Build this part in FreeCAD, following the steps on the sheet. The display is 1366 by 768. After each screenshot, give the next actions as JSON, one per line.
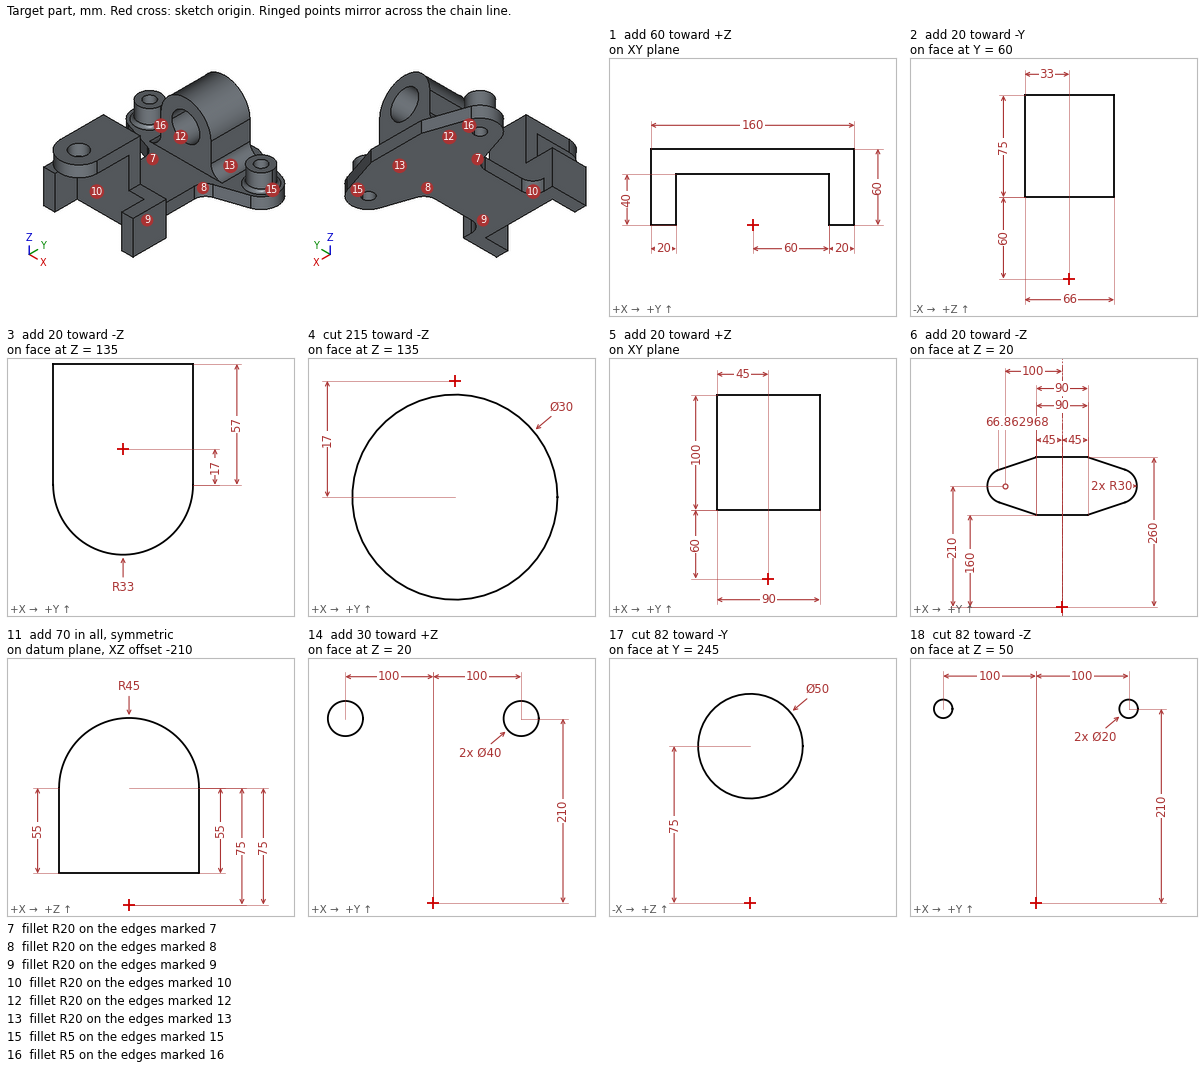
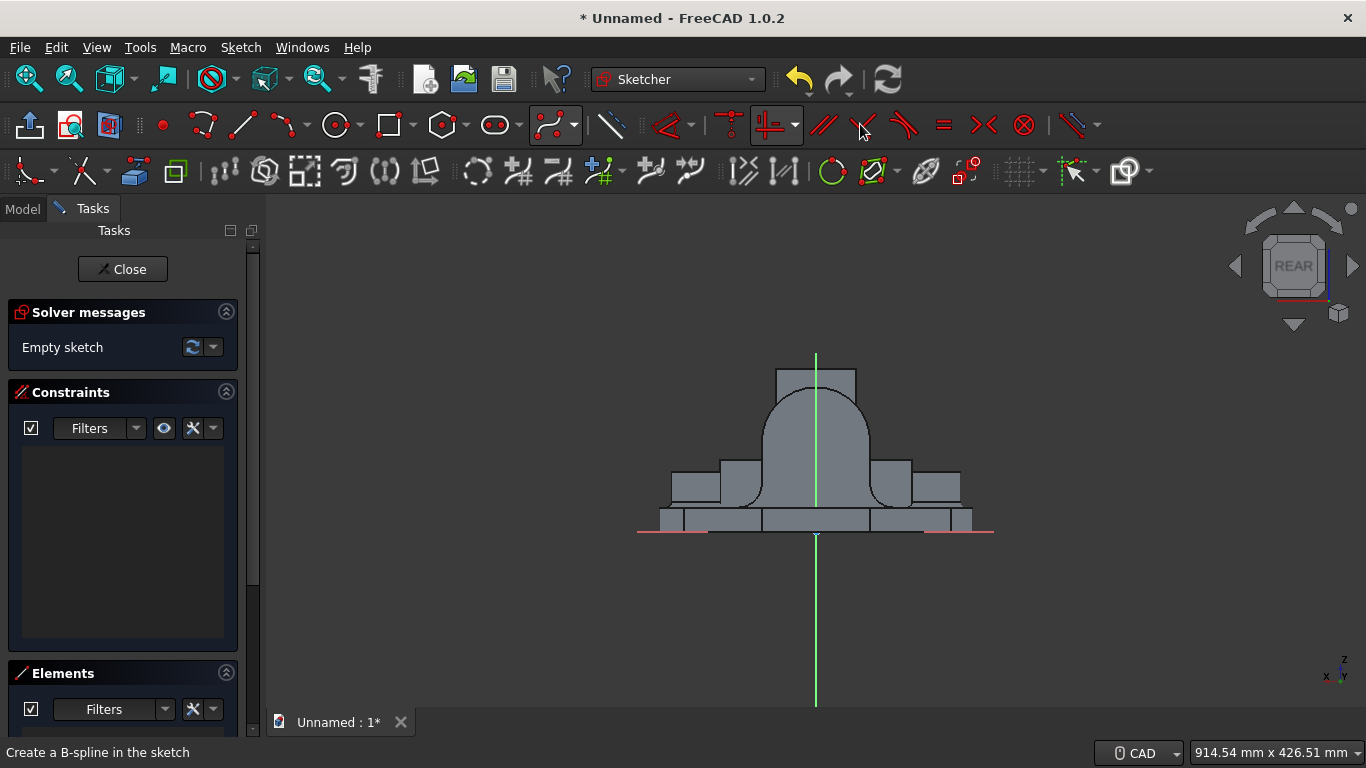
{"action": "left_click", "coordinate": [110, 126]}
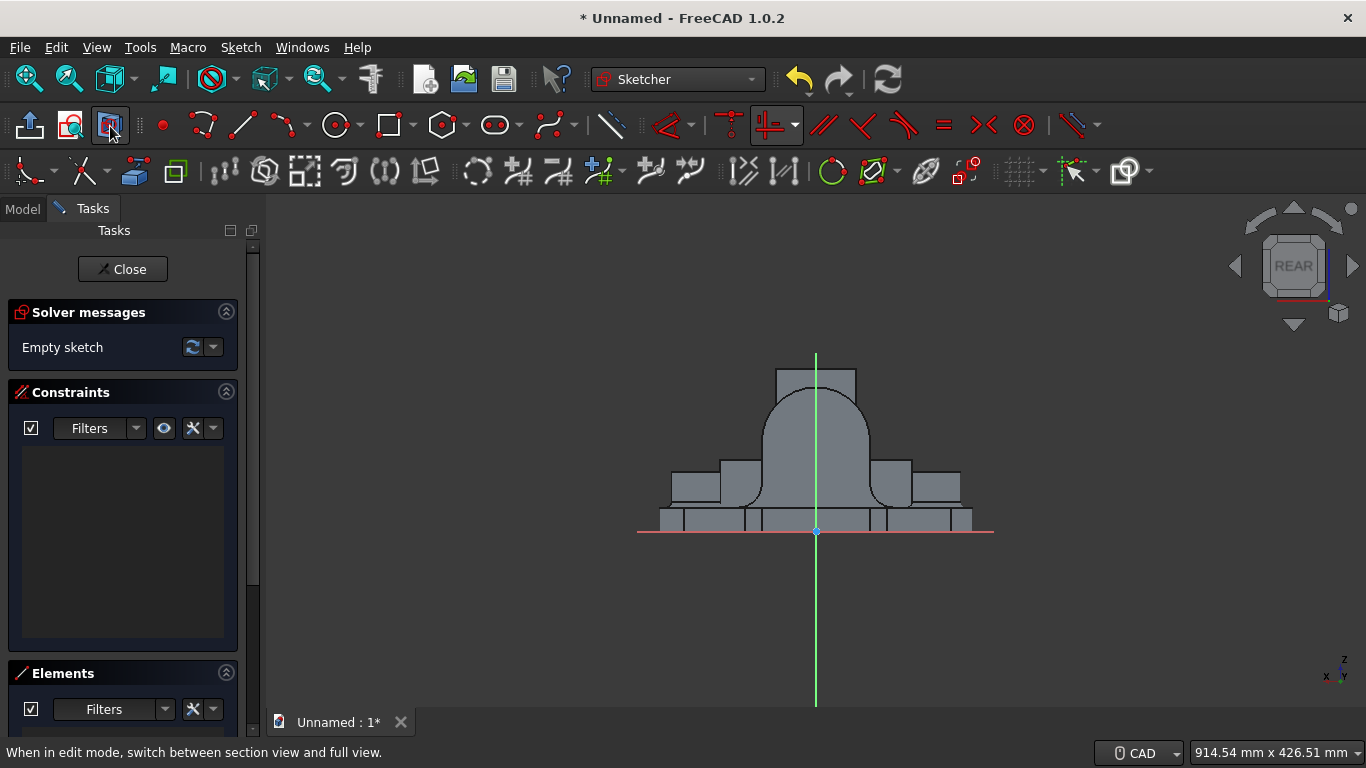
{"action": "scroll", "coordinate": [856, 484], "scroll_direction": "up", "scroll_amount": 5}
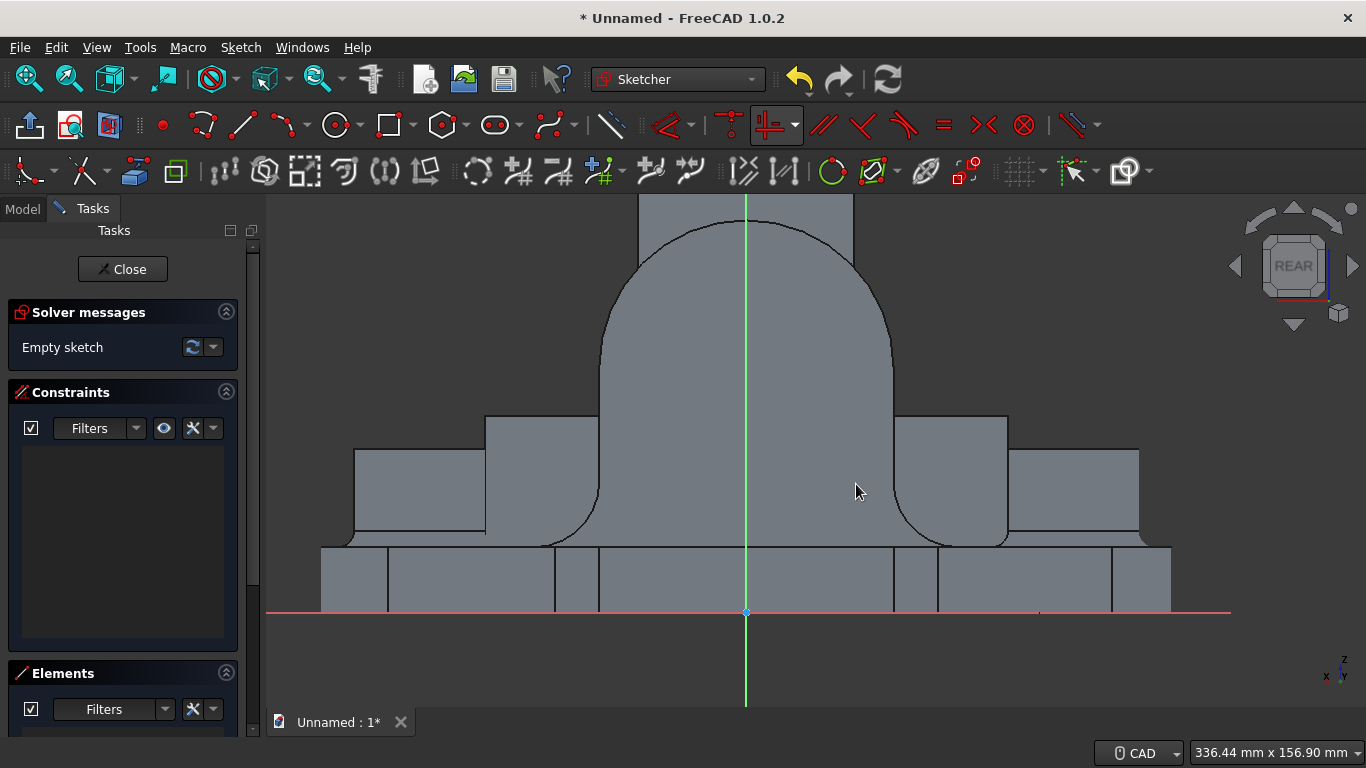
{"action": "key", "text": "g c"}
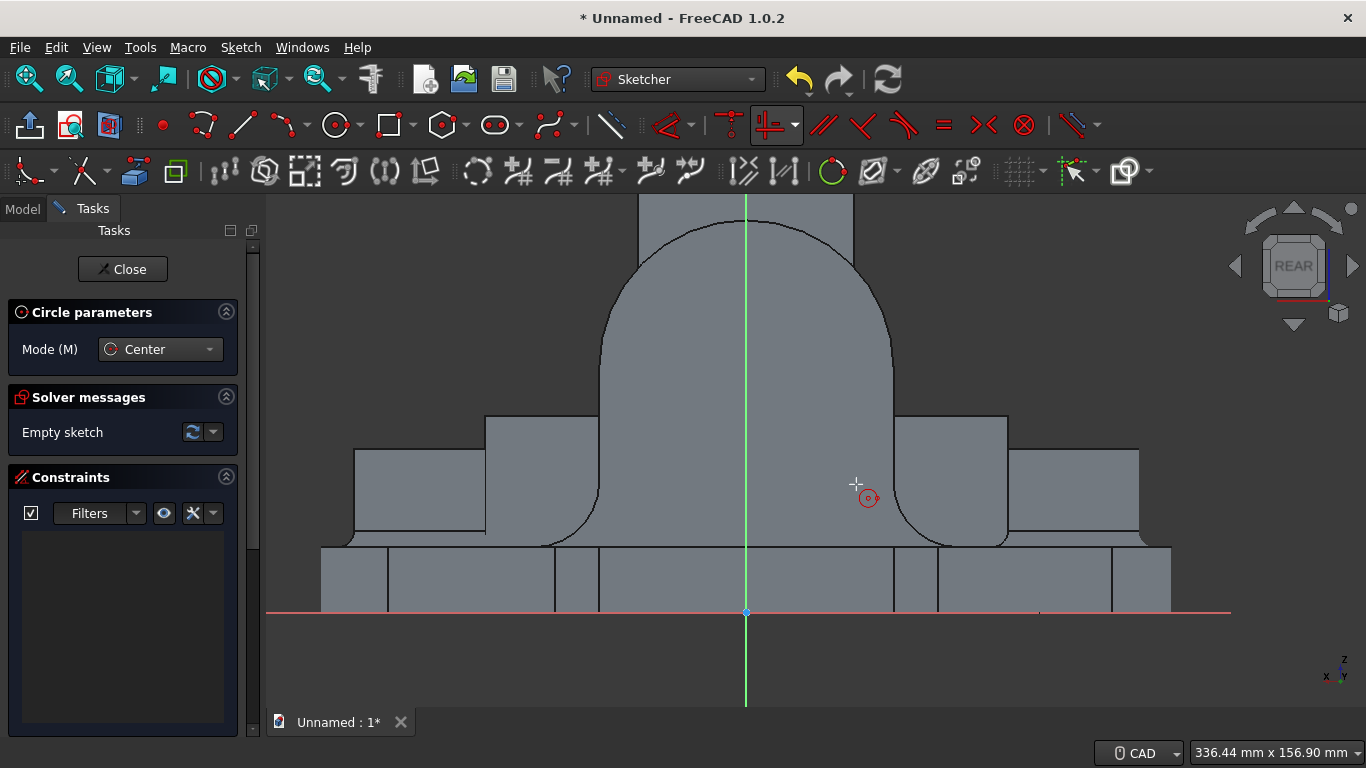
{"action": "left_click", "coordinate": [746, 367]}
{"action": "left_click", "coordinate": [804, 310]}
{"action": "key", "text": "Escape"}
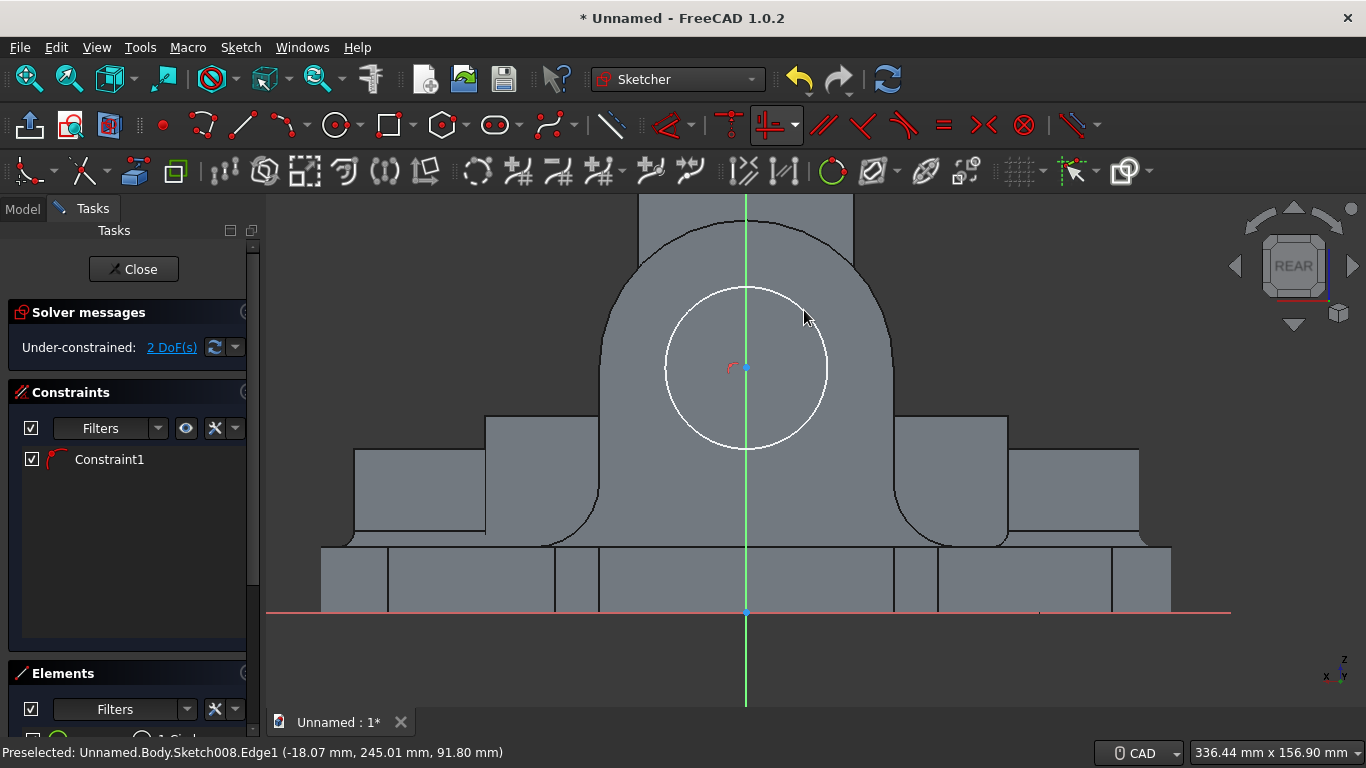
{"action": "key", "text": "d"}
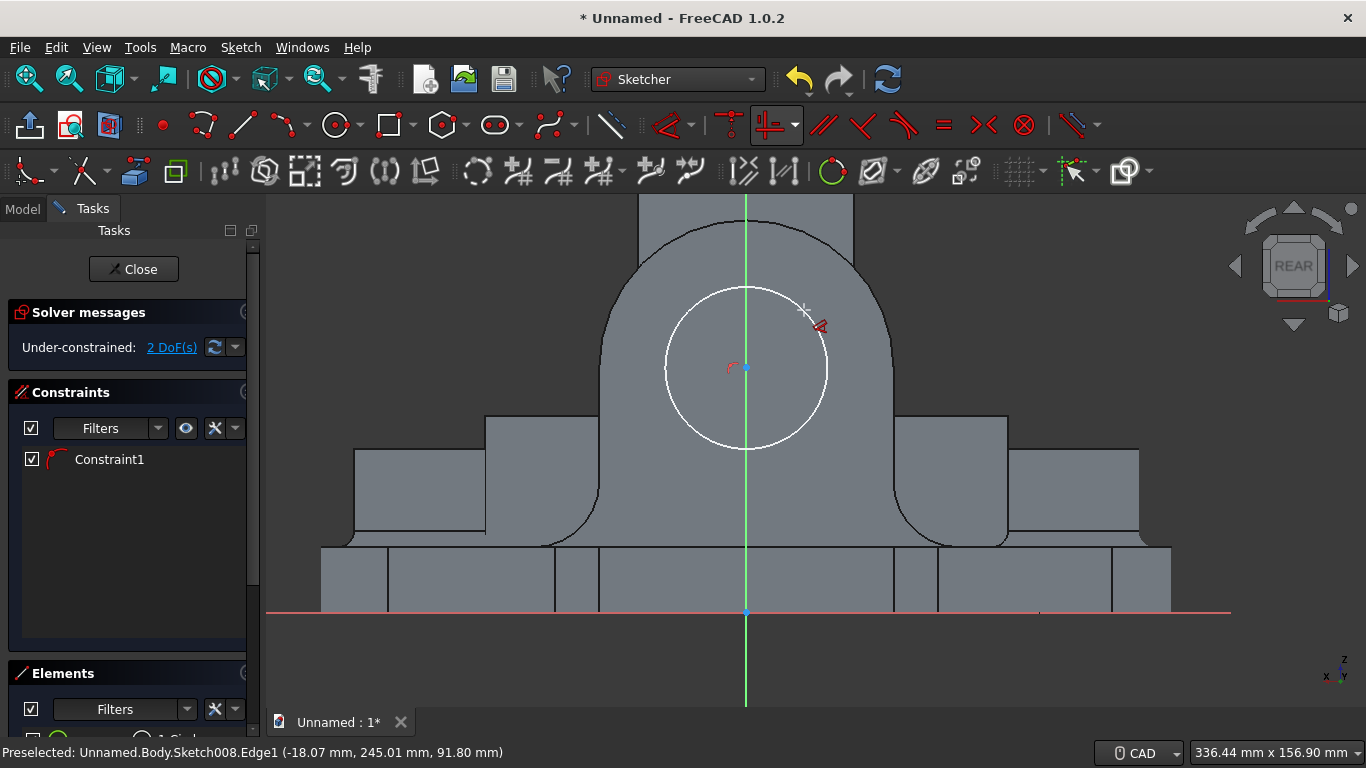
{"action": "left_click", "coordinate": [804, 311]}
{"action": "left_click", "coordinate": [827, 288]}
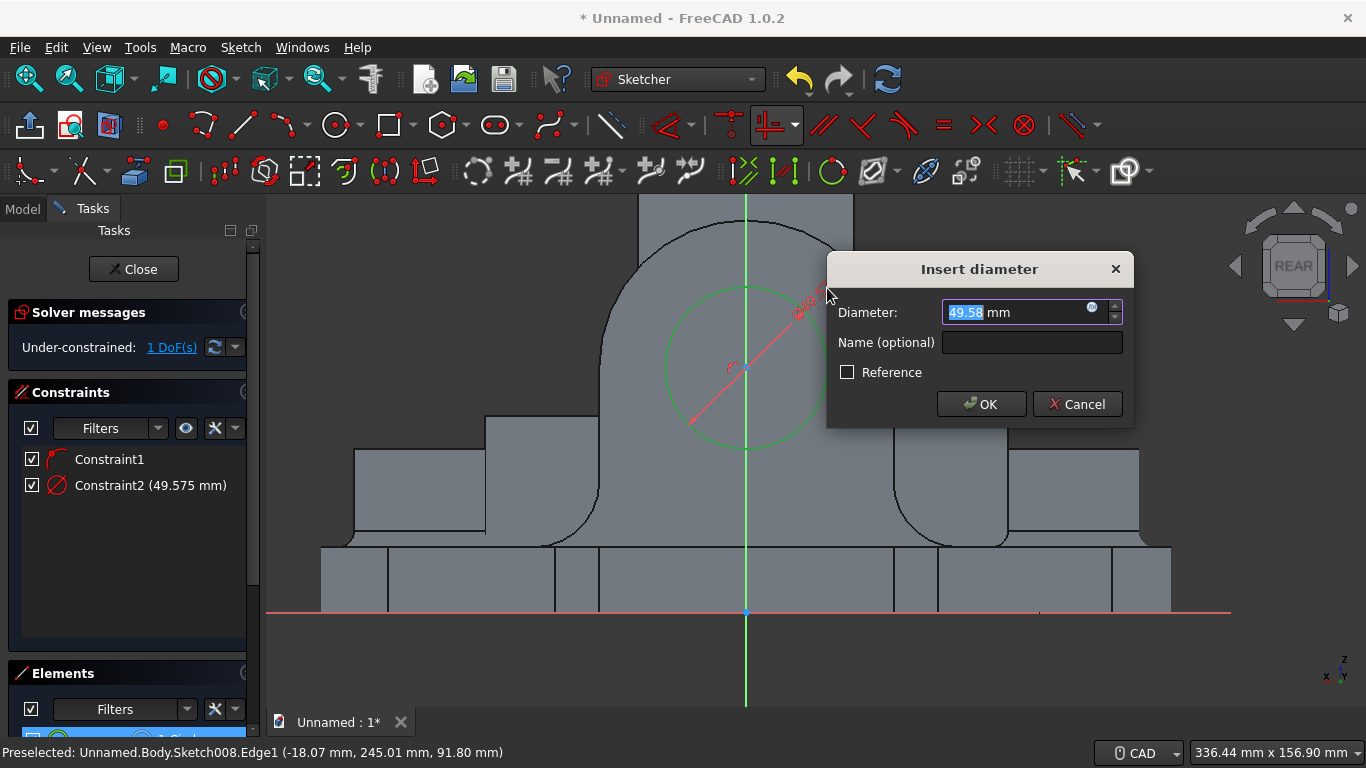
{"action": "type", "text": "50"}
{"action": "key", "text": "Return"}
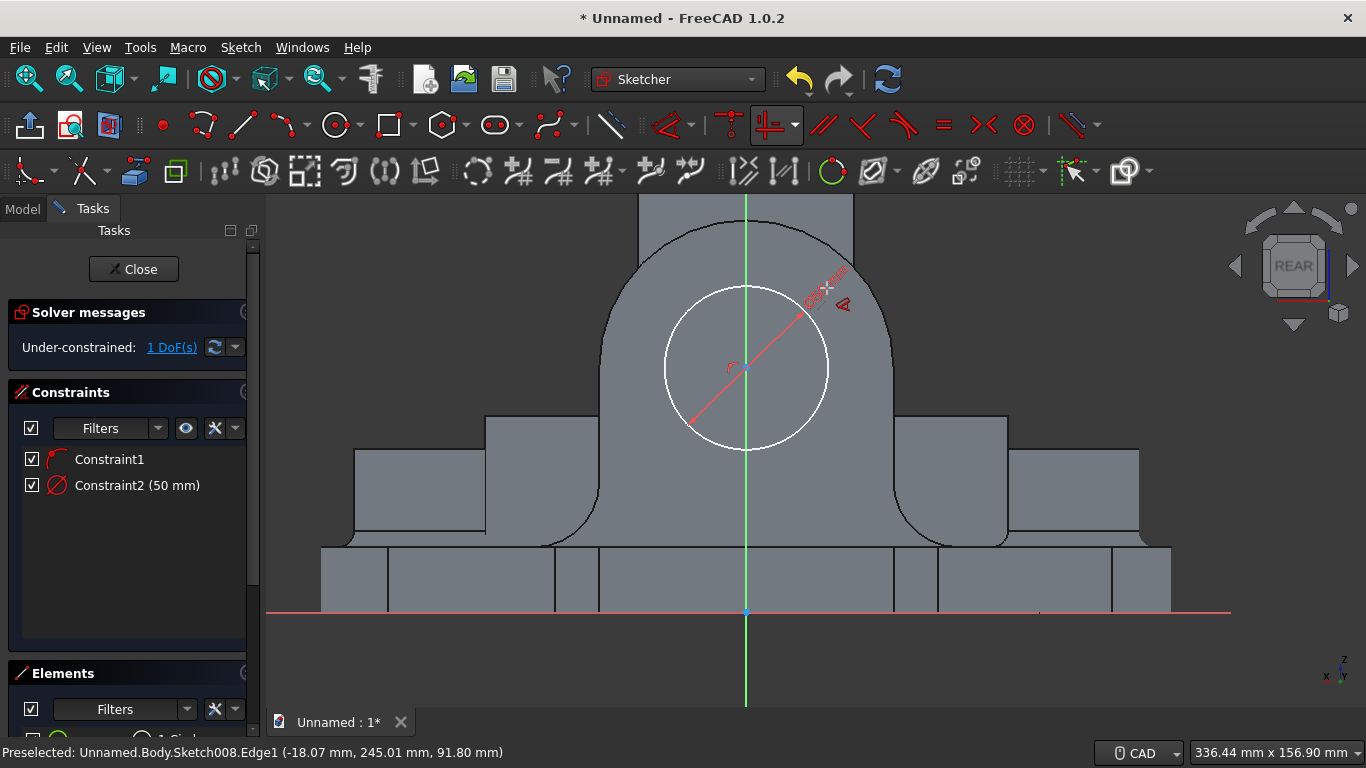
{"action": "left_click", "coordinate": [746, 368]}
{"action": "left_click", "coordinate": [780, 490]}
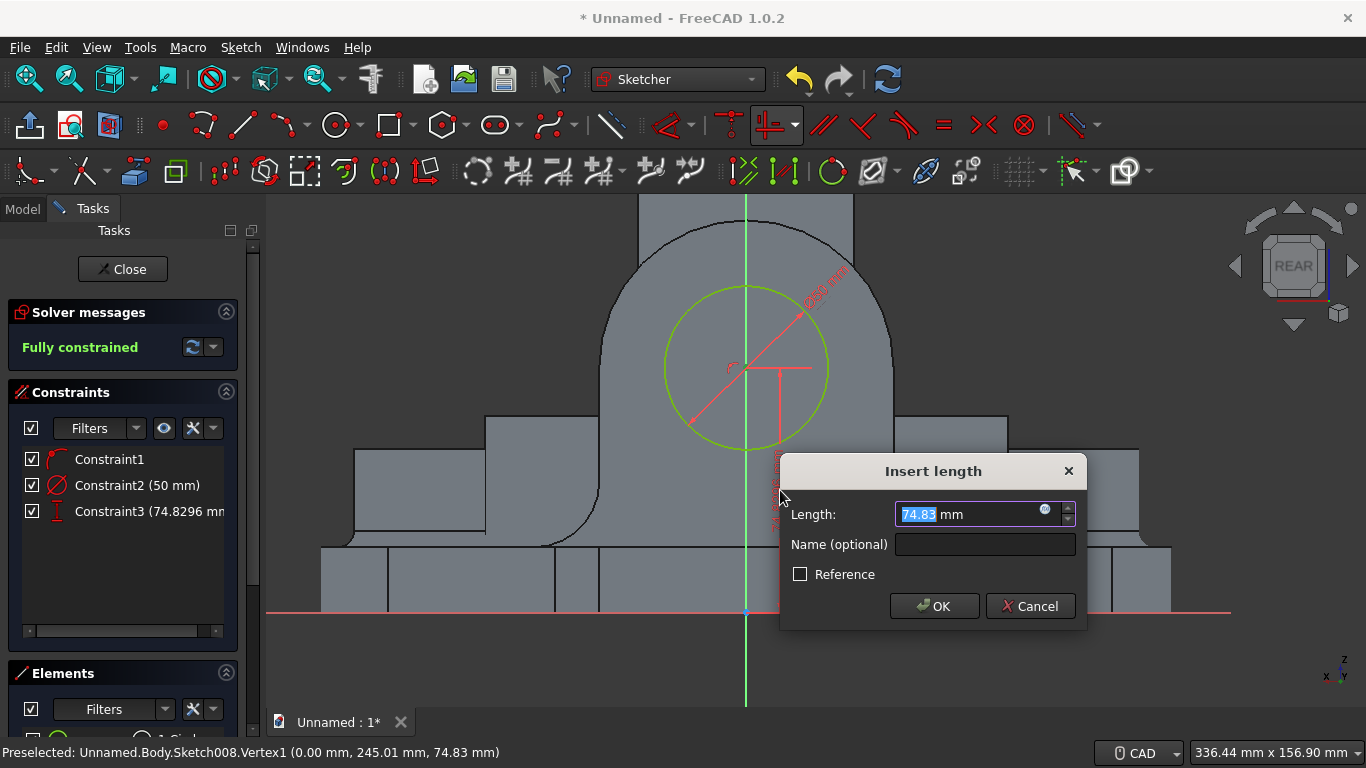
{"action": "type", "text": "75"}
{"action": "key", "text": "Return"}
{"action": "key", "text": "Escape"}